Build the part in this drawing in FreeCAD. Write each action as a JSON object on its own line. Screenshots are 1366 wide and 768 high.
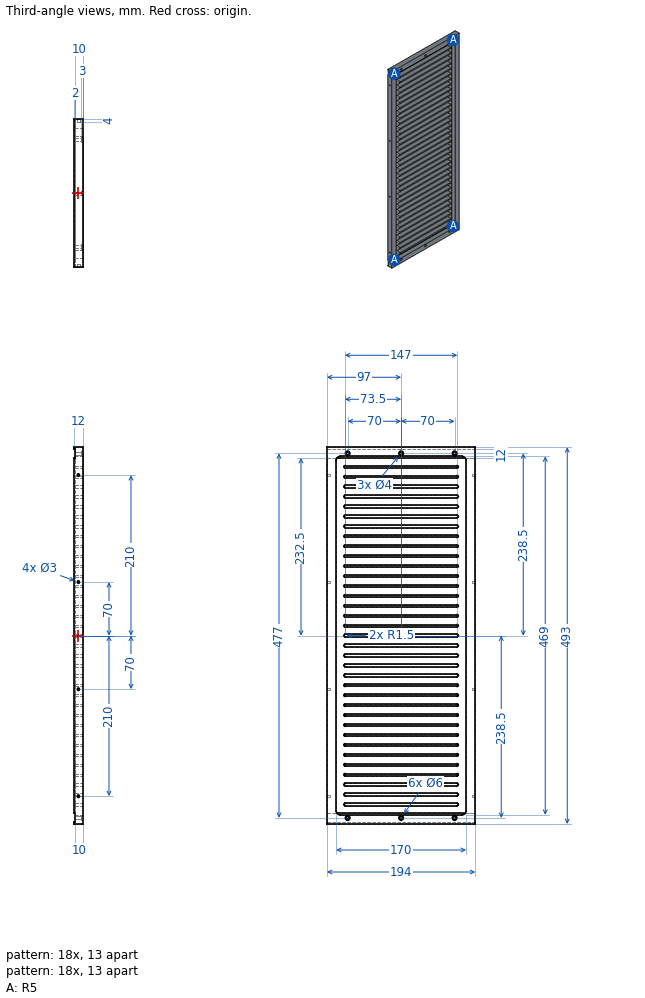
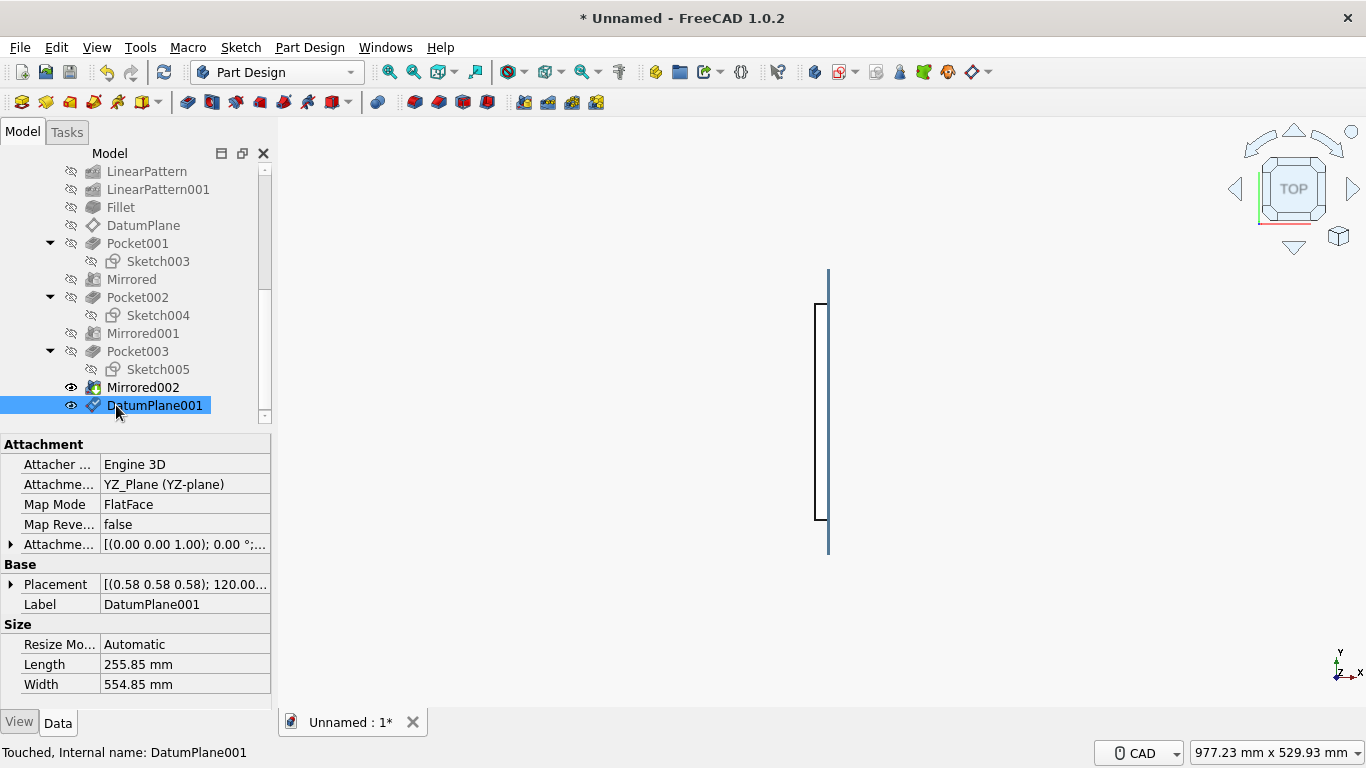
{"action": "left_click", "coordinate": [840, 72]}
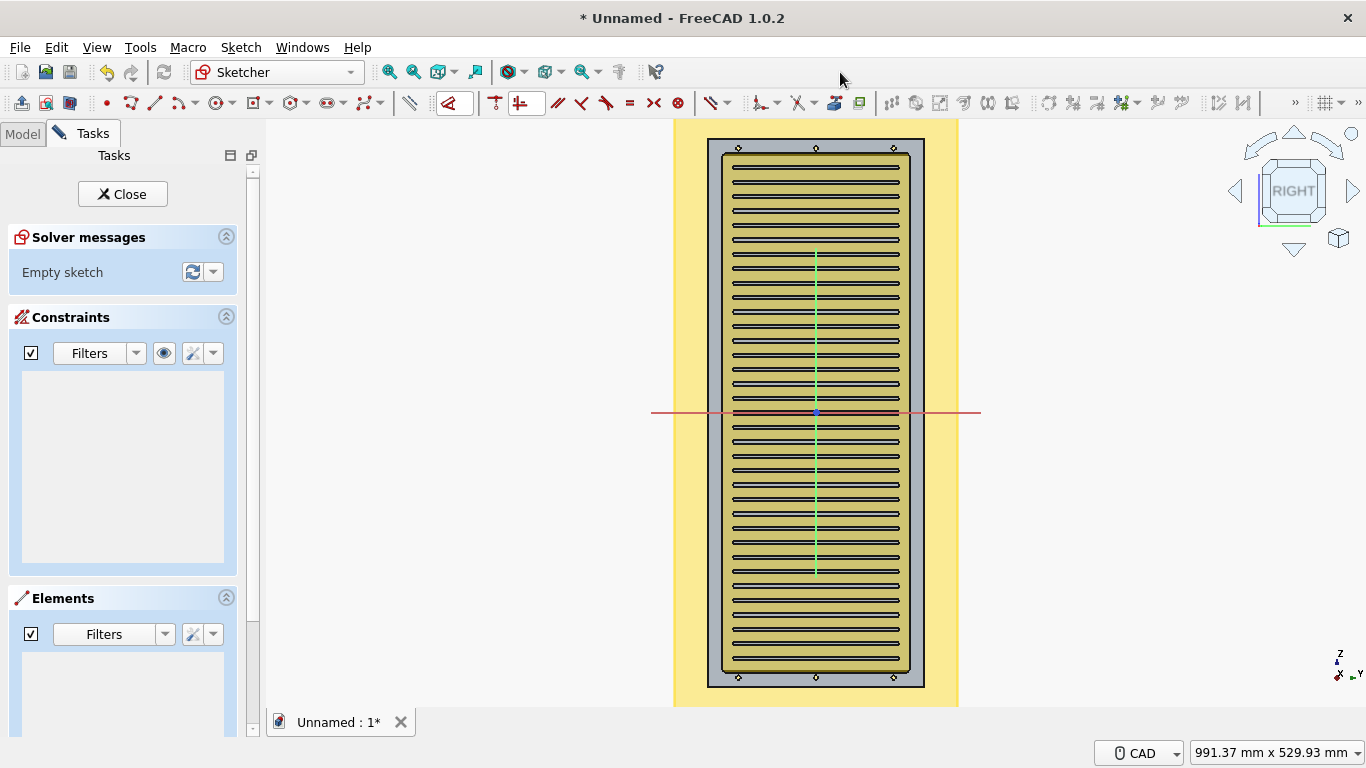
{"action": "scroll", "coordinate": [608, 413], "scroll_direction": "down", "scroll_amount": 2}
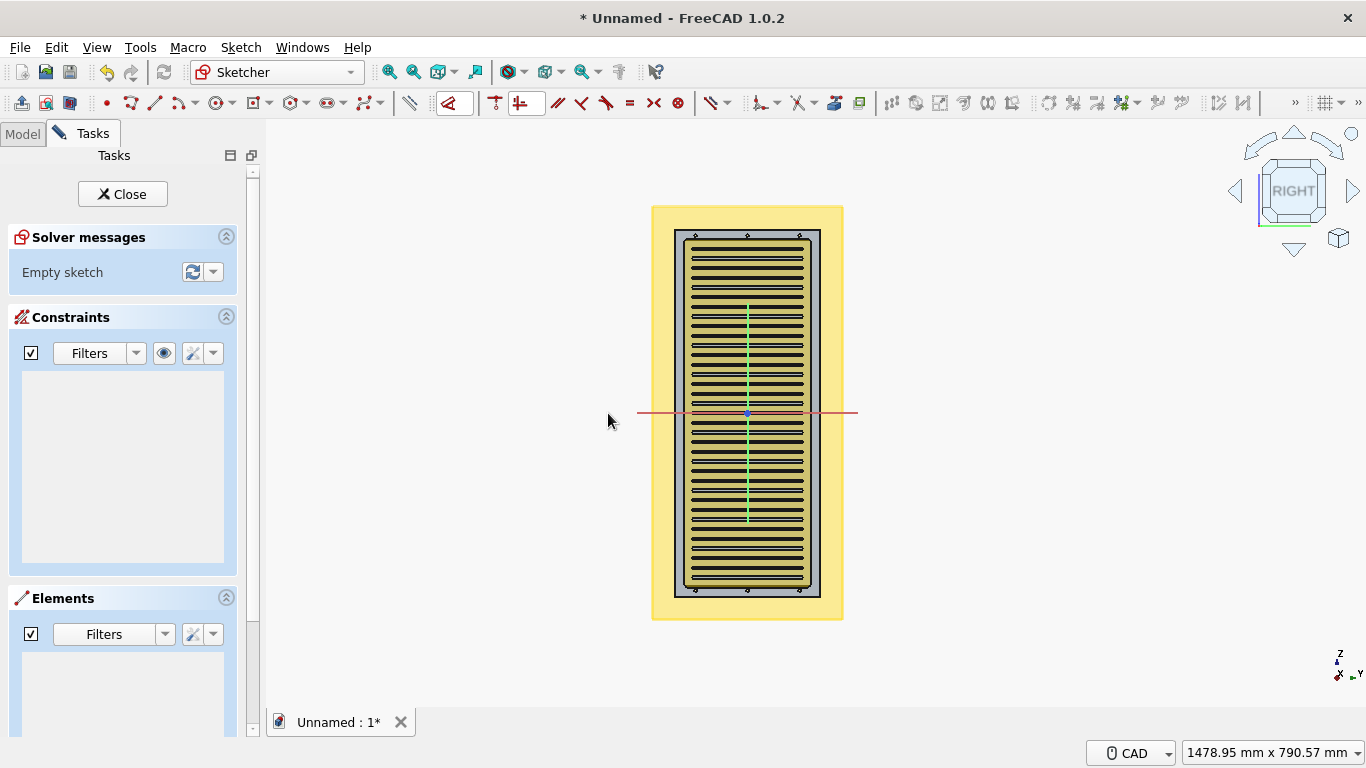
{"action": "left_click", "coordinate": [216, 104]}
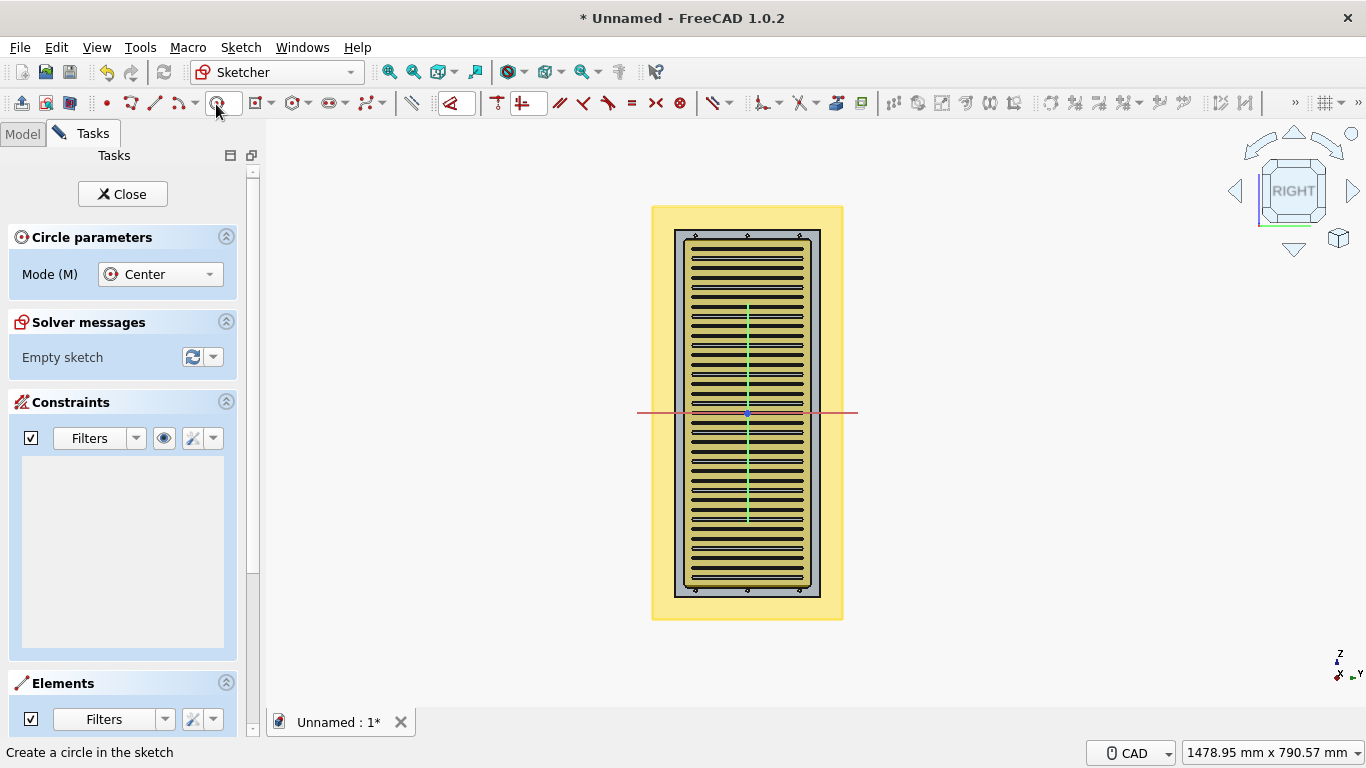
{"action": "scroll", "coordinate": [748, 591], "scroll_direction": "up", "scroll_amount": 12}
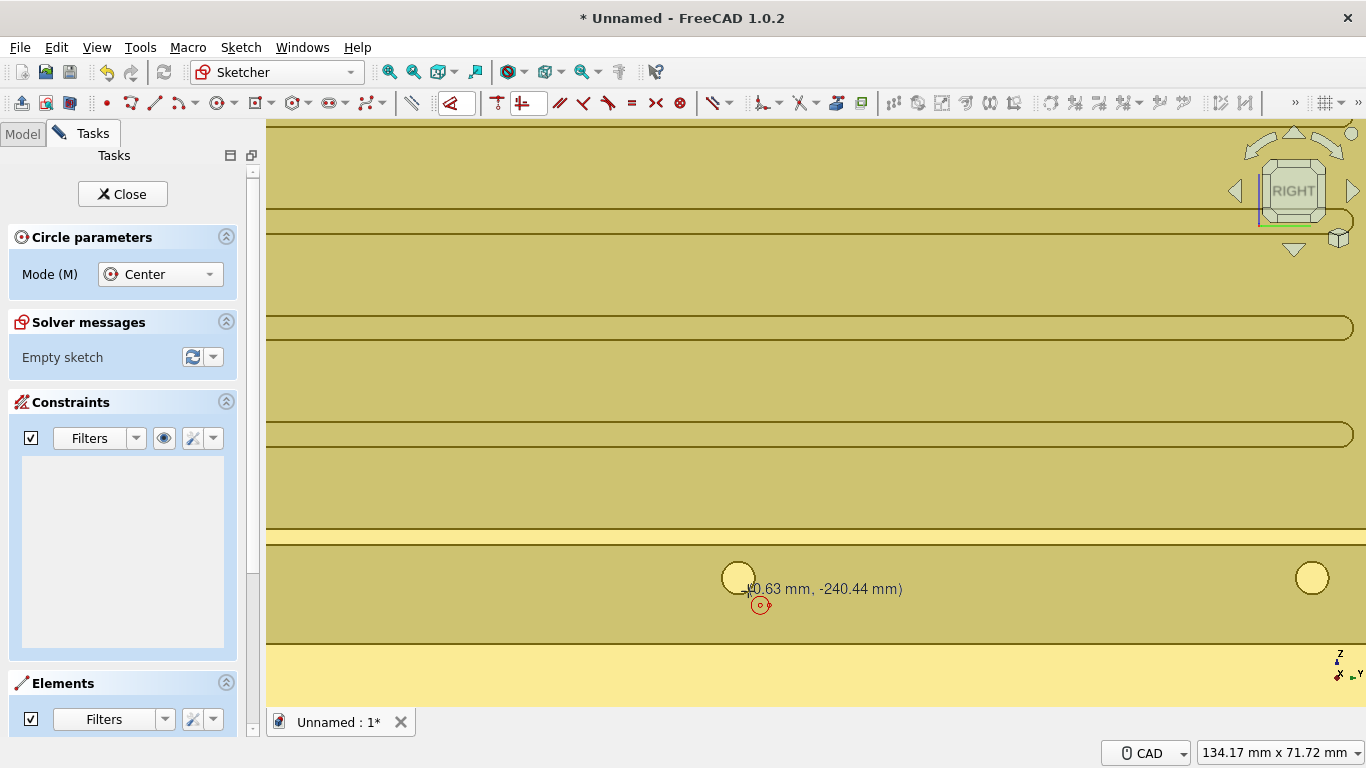
{"action": "scroll", "coordinate": [748, 592], "scroll_direction": "down", "scroll_amount": 12}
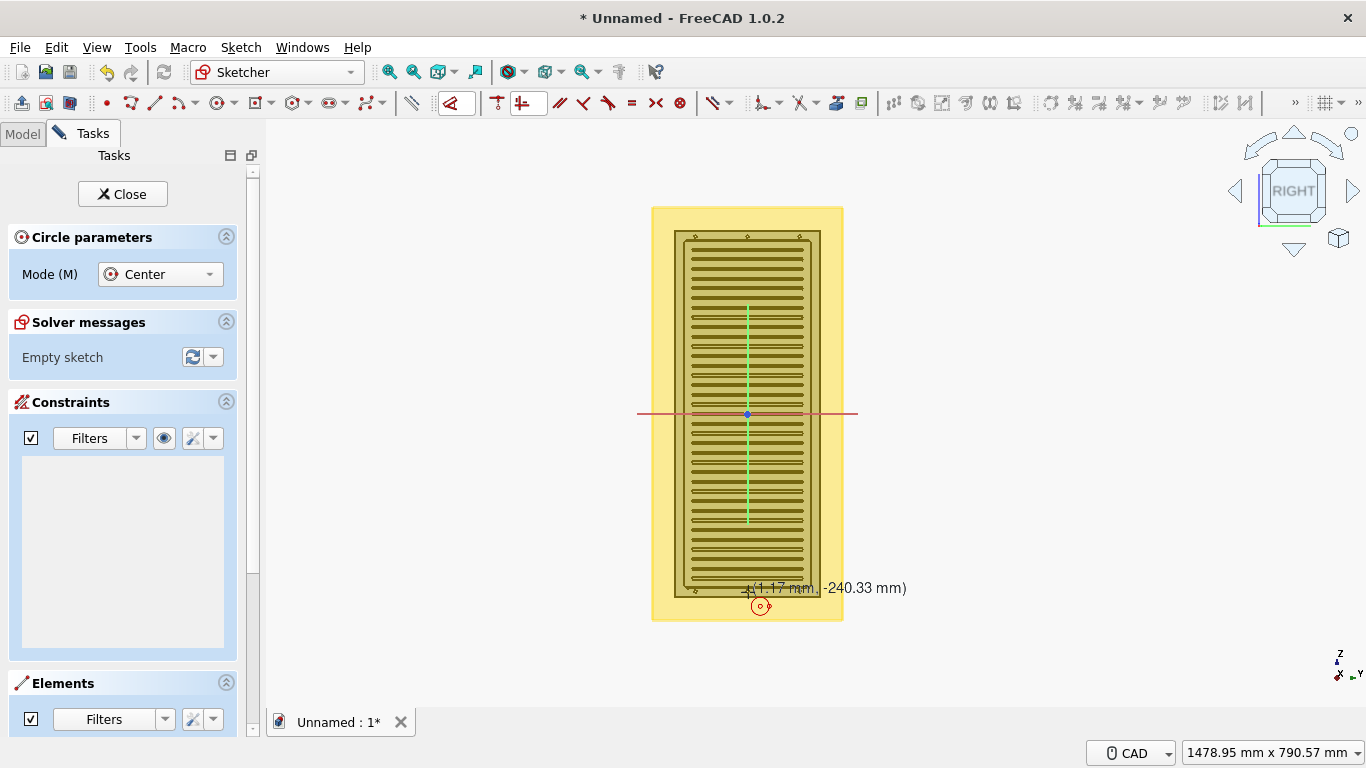
{"action": "left_click", "coordinate": [748, 591]}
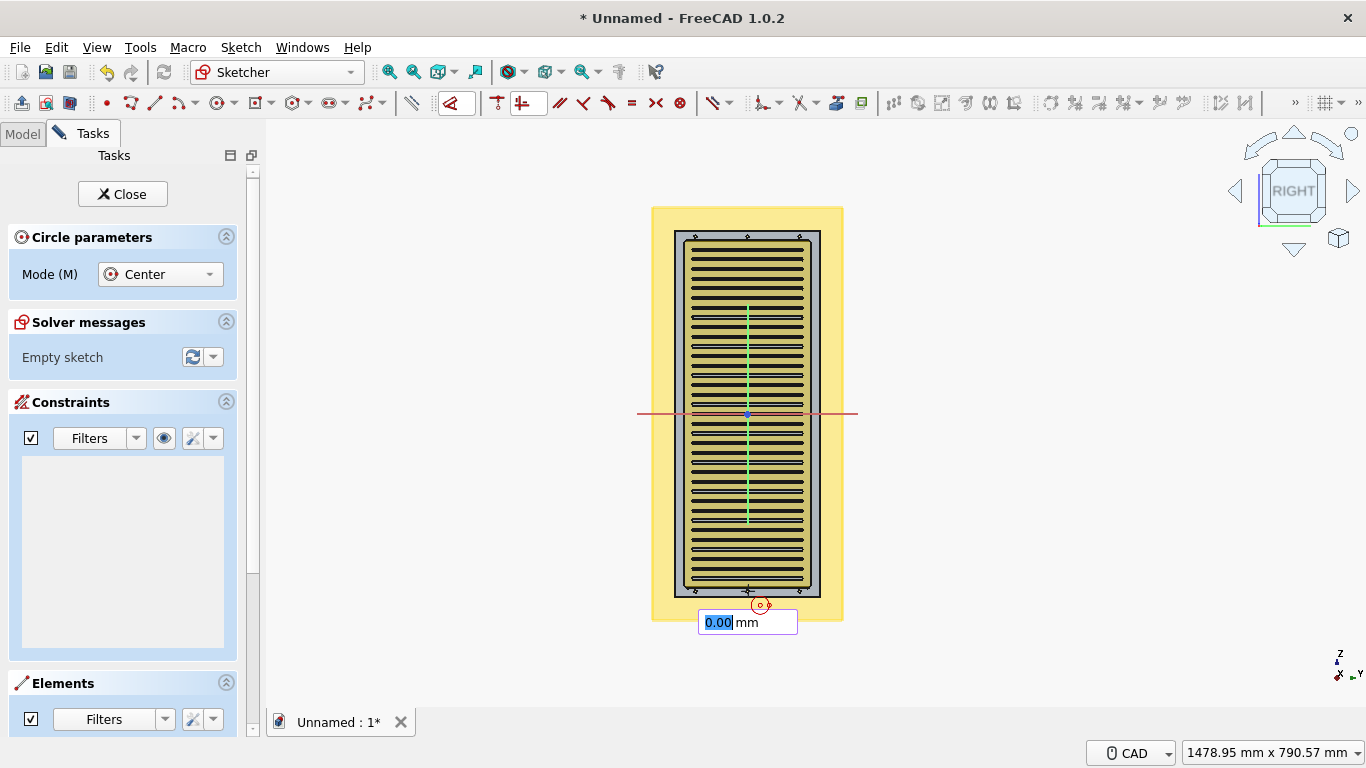
{"action": "scroll", "coordinate": [750, 591], "scroll_direction": "up", "scroll_amount": 11}
{"action": "mouse_move", "coordinate": [743, 582]}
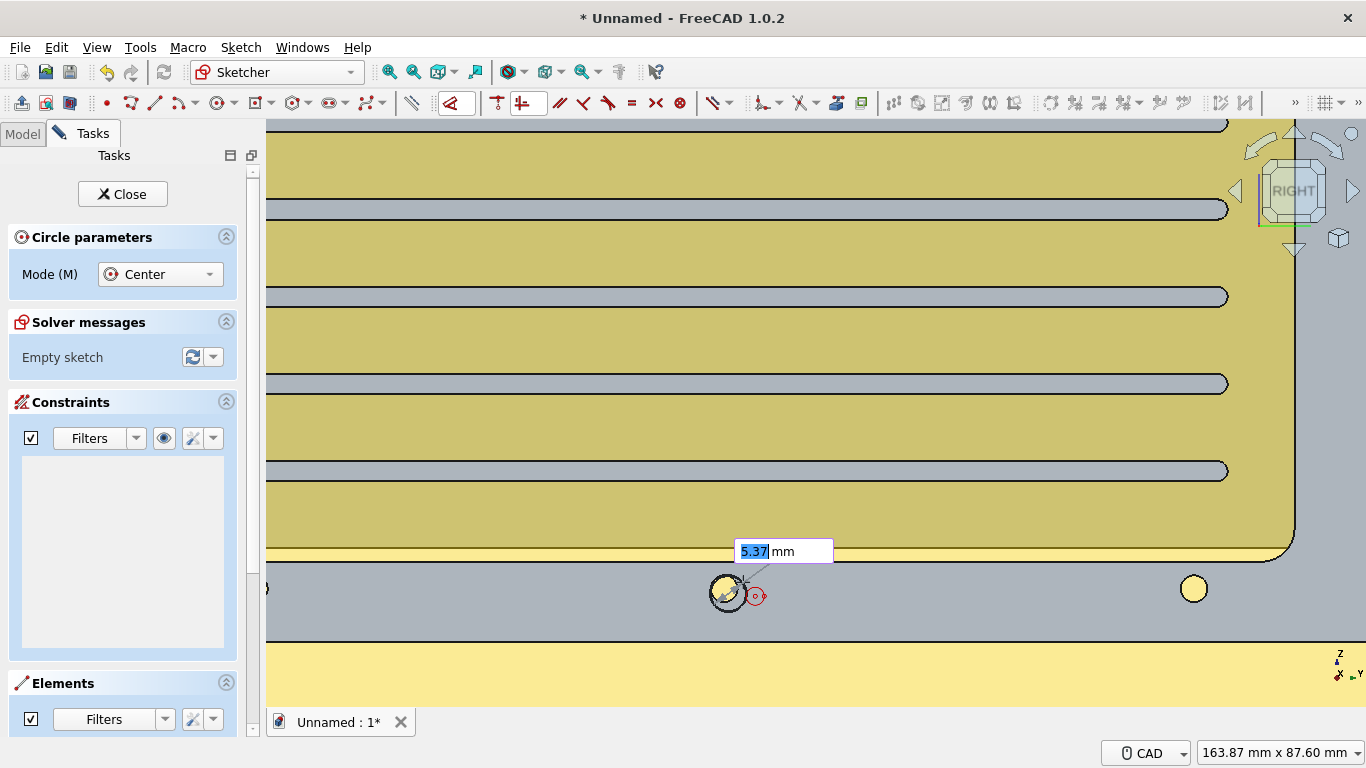
{"action": "type", "text": "6"}
{"action": "key", "text": "Return"}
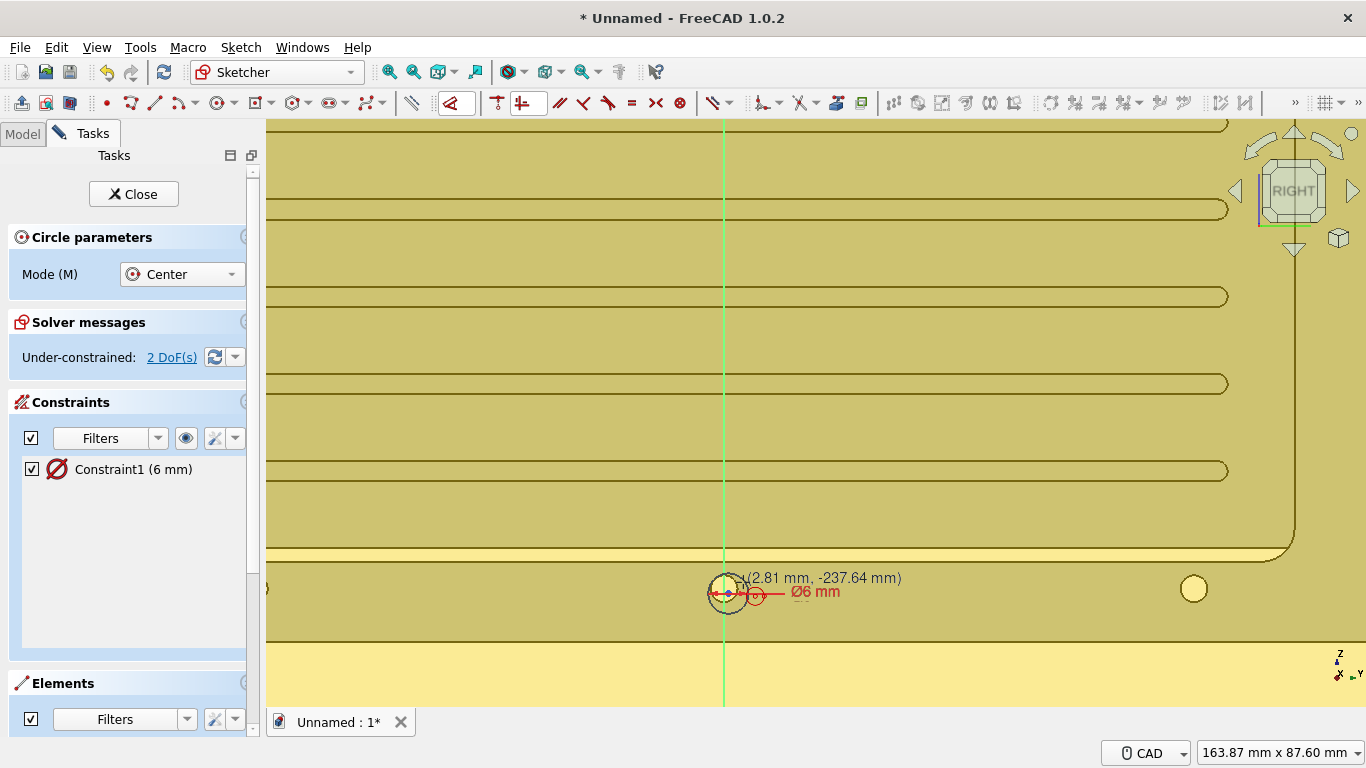
{"action": "scroll", "coordinate": [750, 591], "scroll_direction": "down", "scroll_amount": 11}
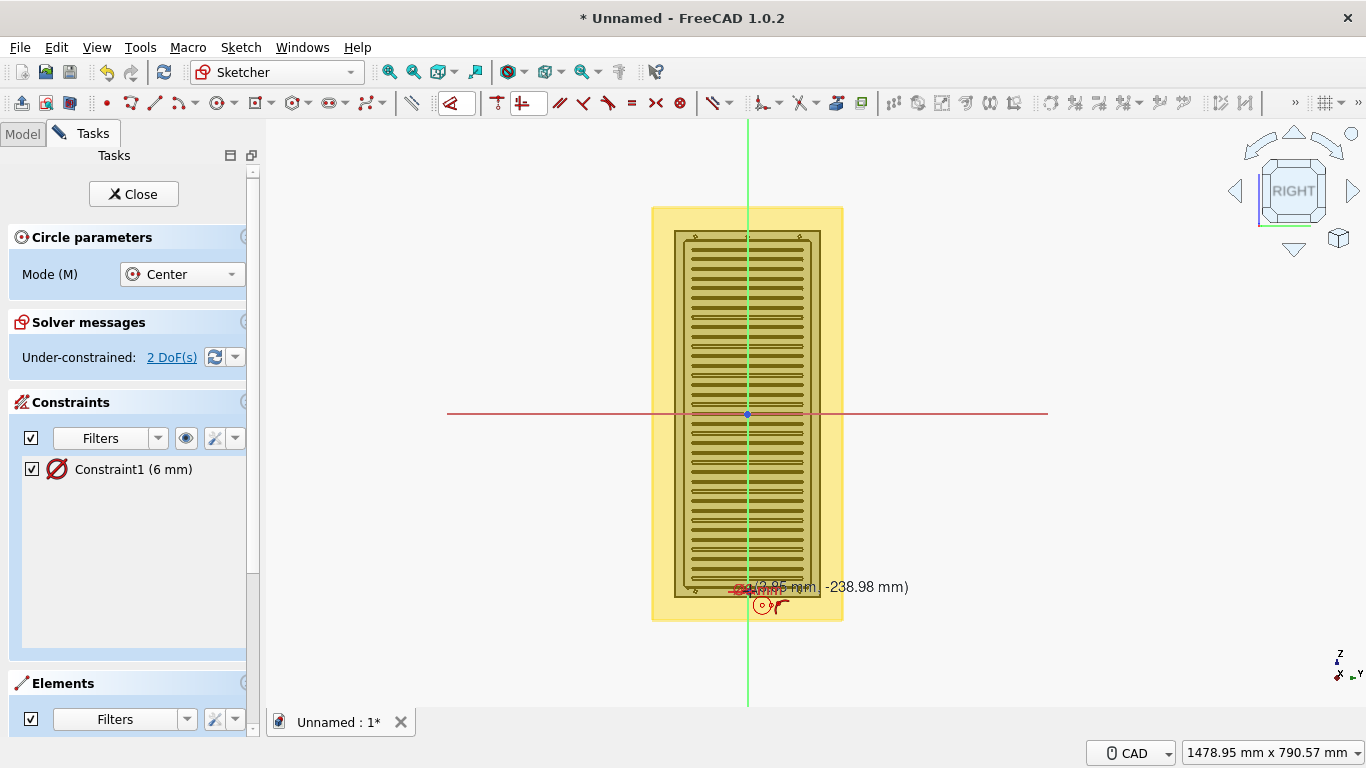
{"action": "left_click", "coordinate": [800, 591]}
{"action": "mouse_move", "coordinate": [801, 590]}